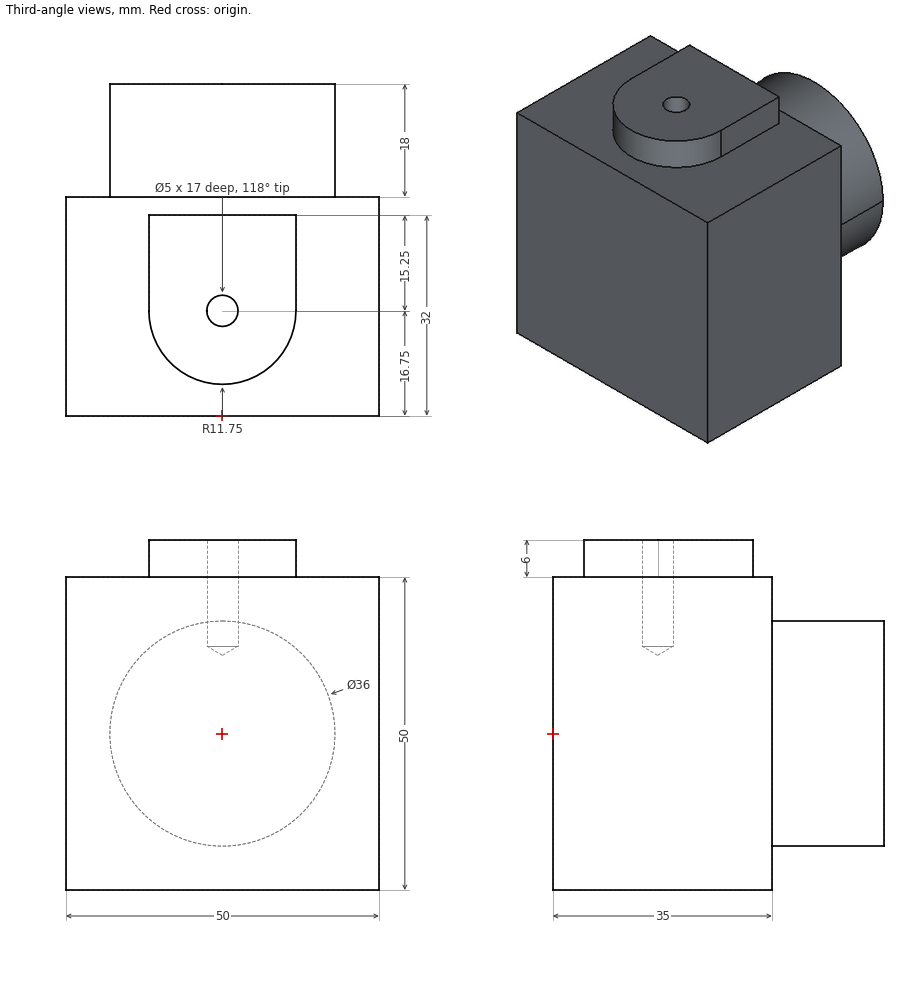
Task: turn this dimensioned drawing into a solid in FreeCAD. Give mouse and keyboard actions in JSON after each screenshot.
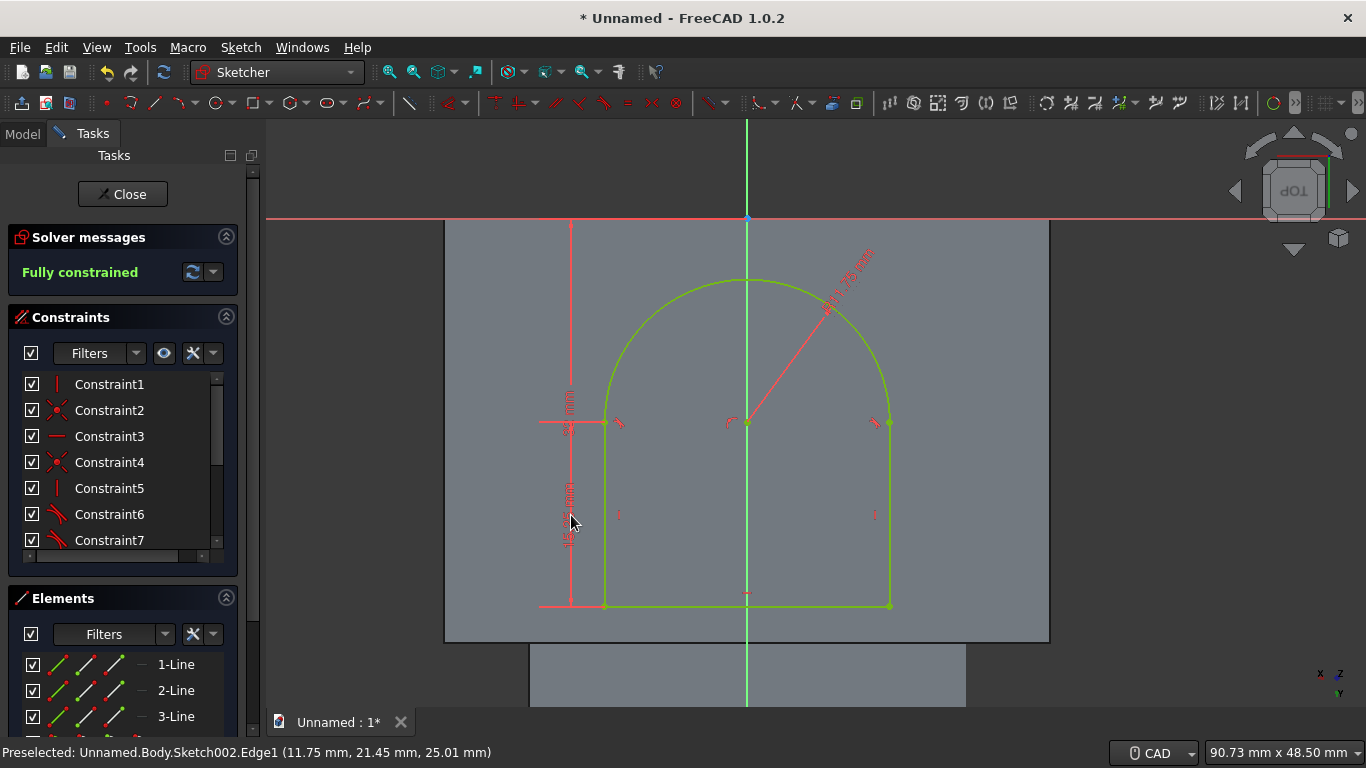
{"action": "left_click", "coordinate": [123, 194]}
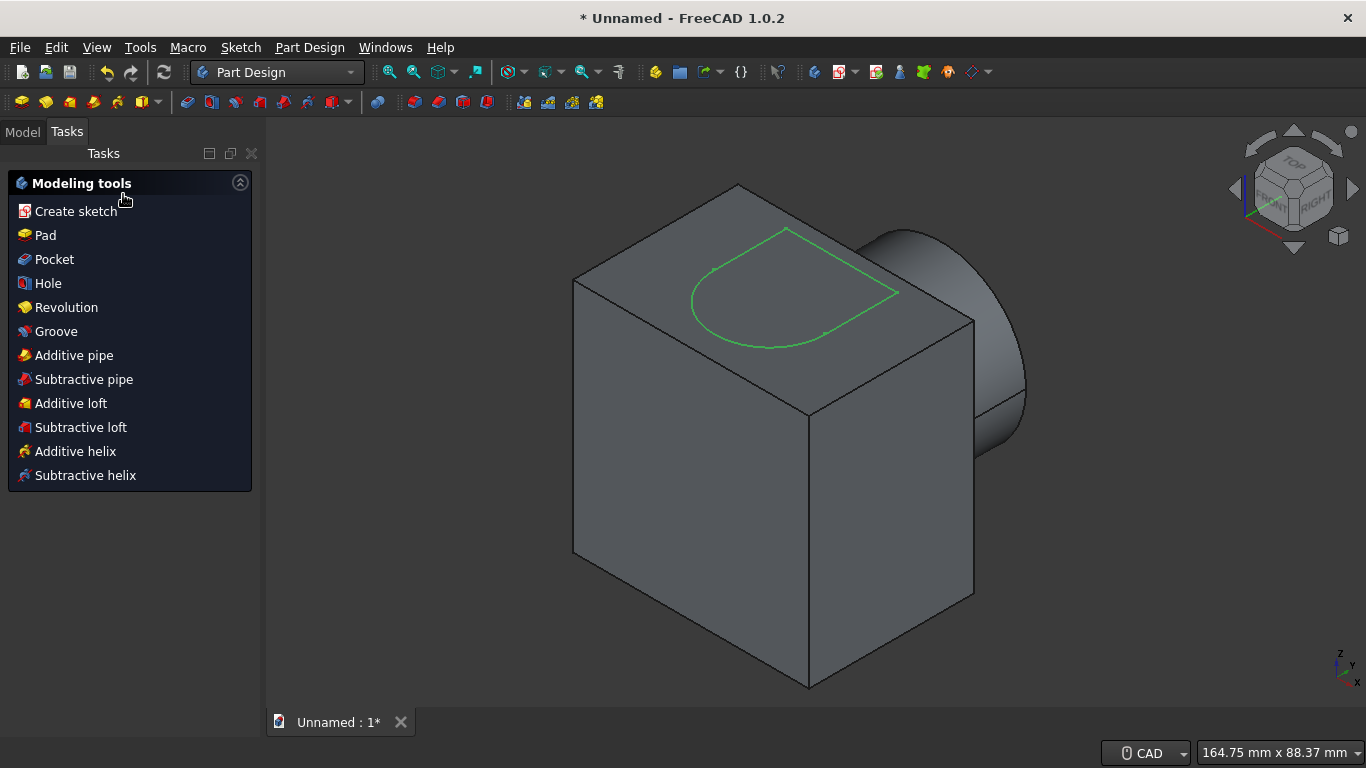
{"action": "left_click", "coordinate": [22, 102]}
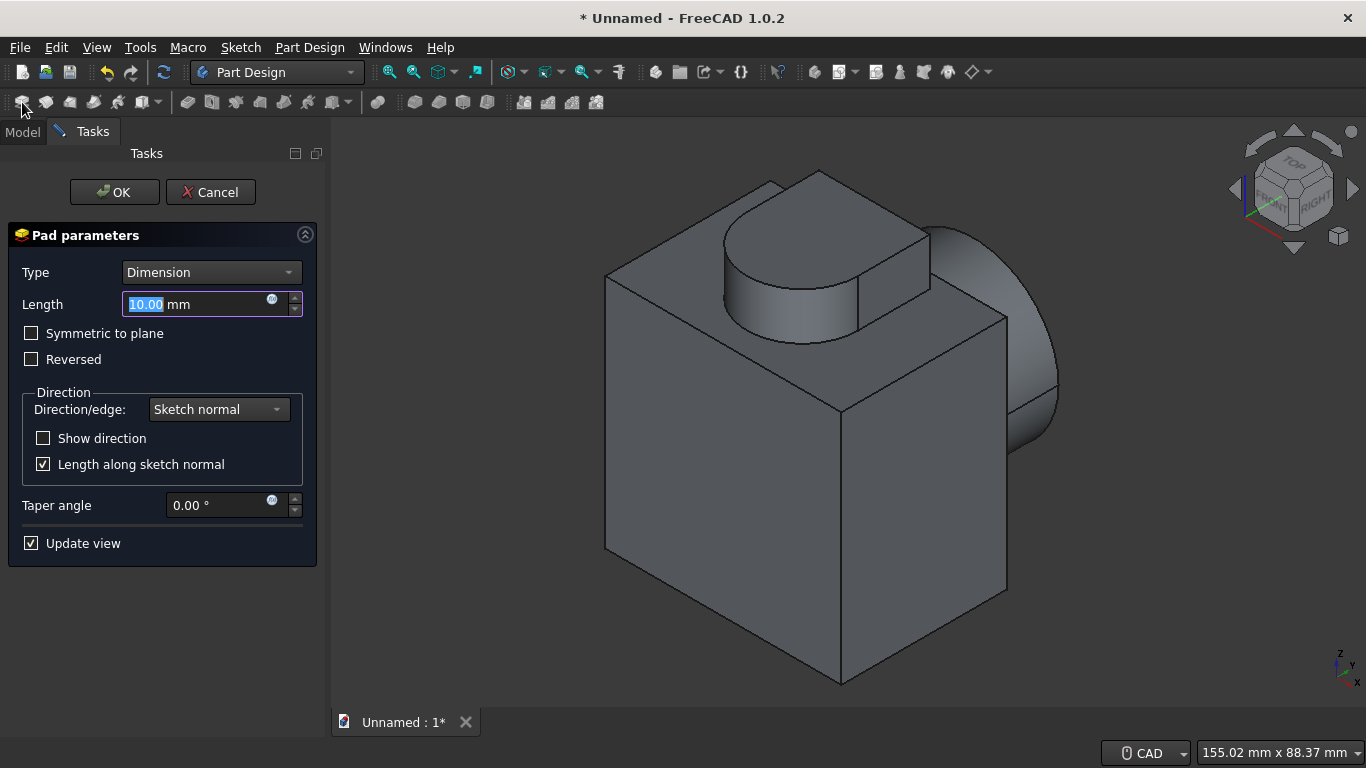
{"action": "type", "text": "6"}
{"action": "key", "text": "Tab"}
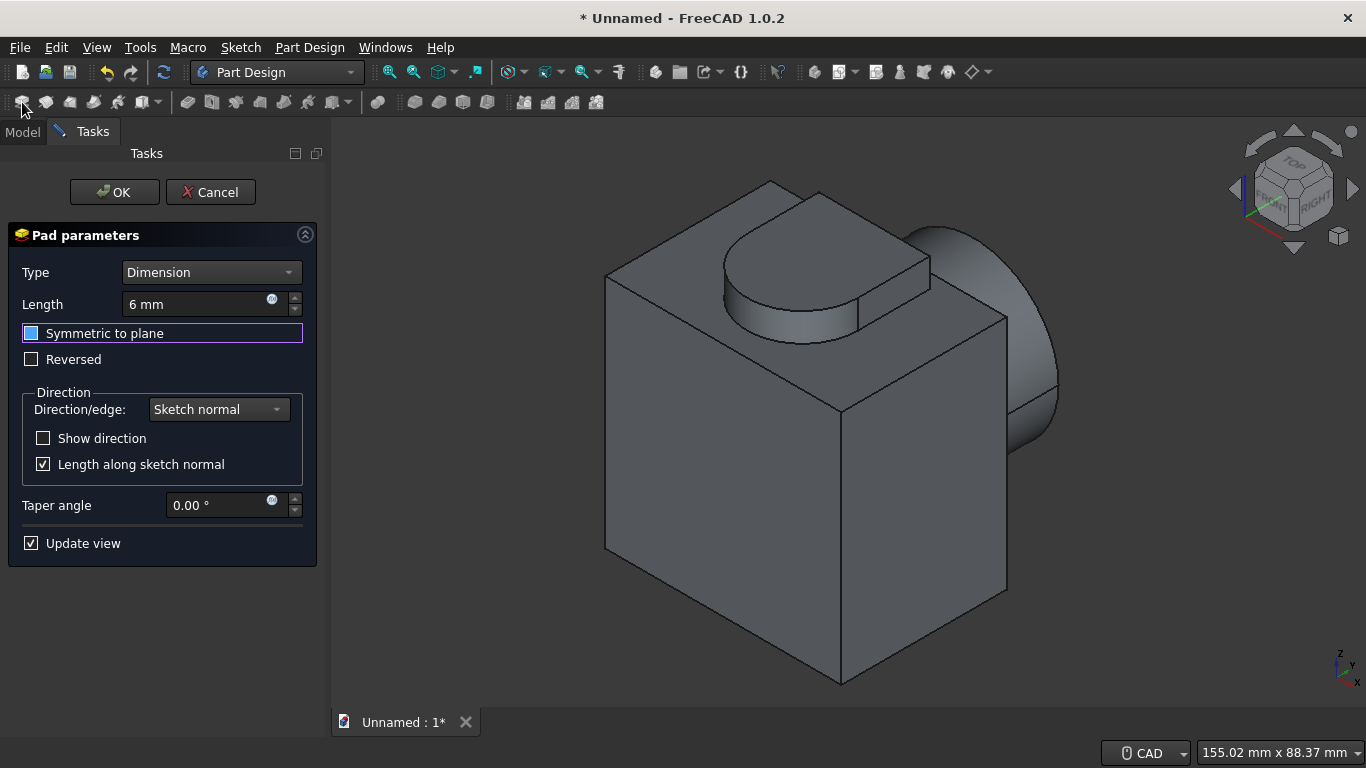
{"action": "left_click", "coordinate": [115, 192]}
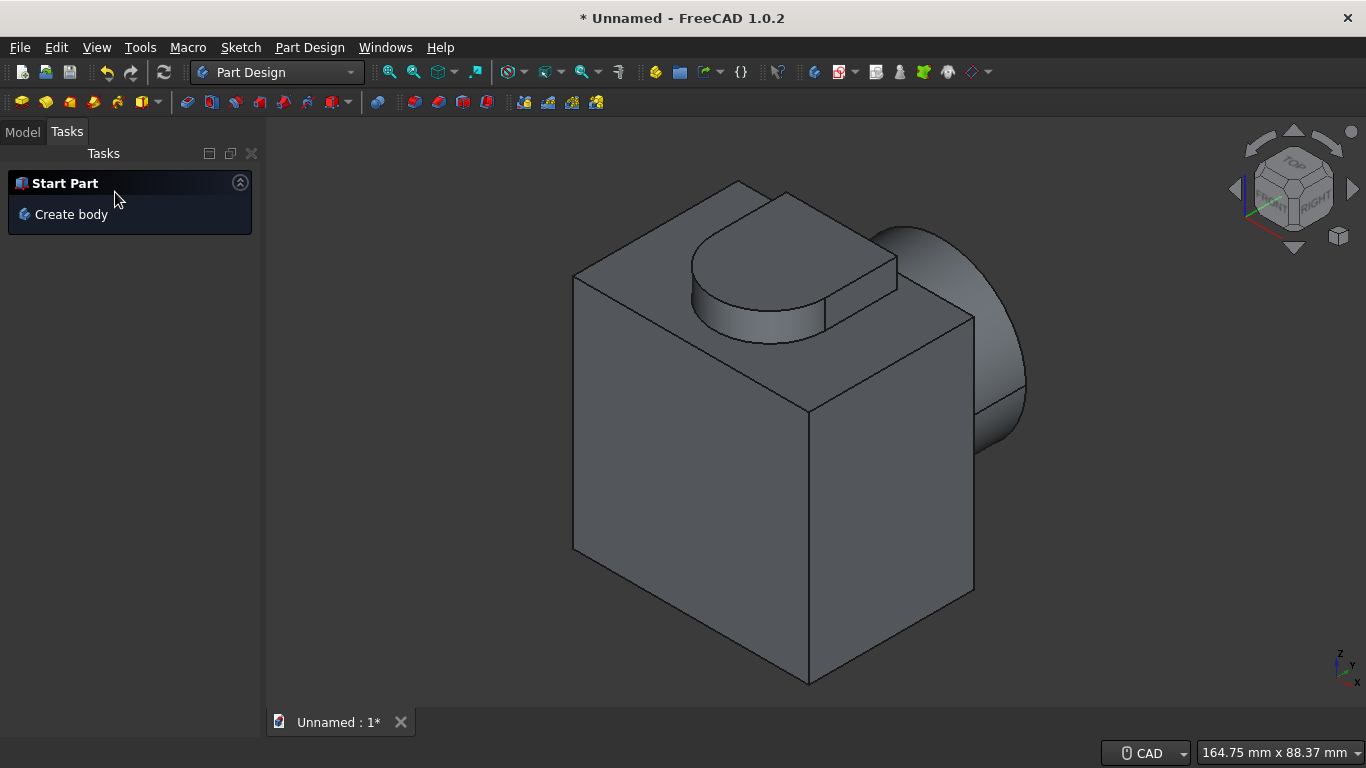
{"action": "left_click", "coordinate": [390, 72]}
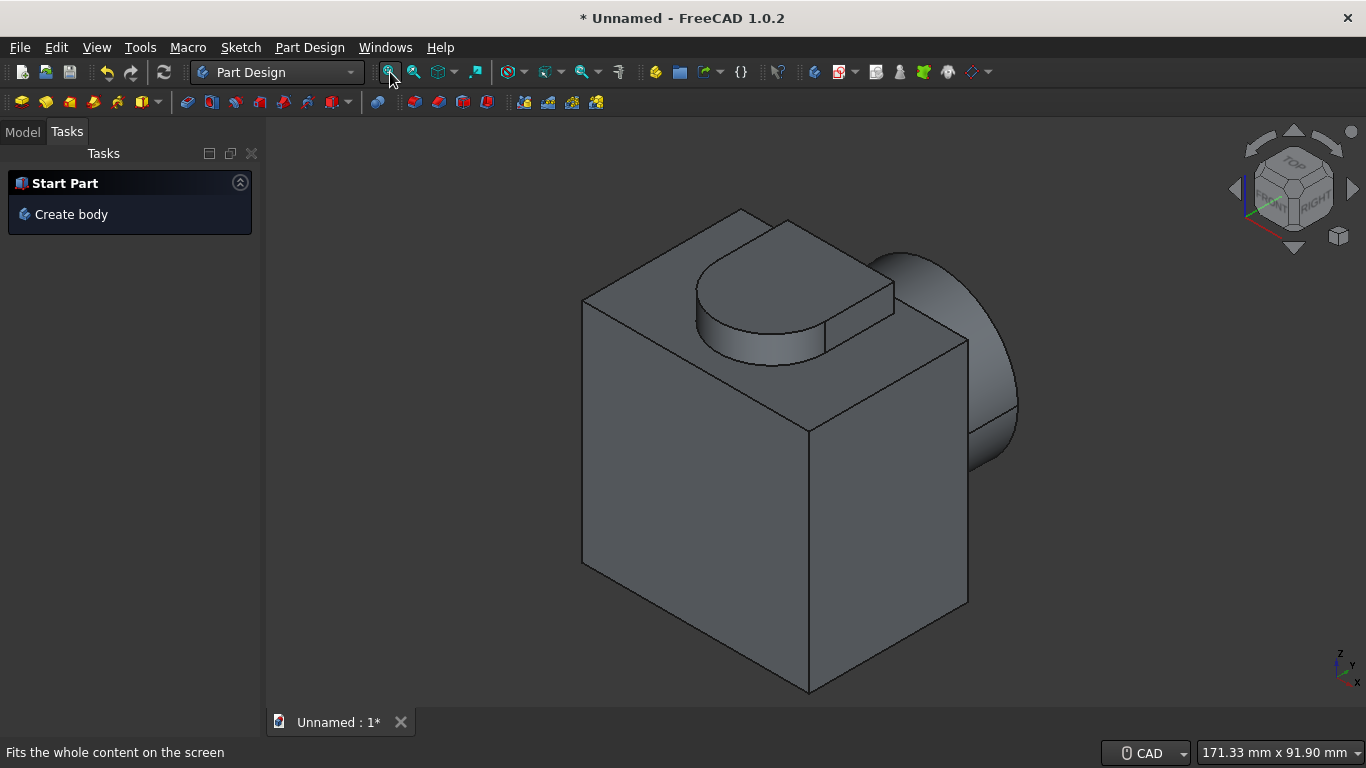
{"action": "left_click", "coordinate": [780, 285]}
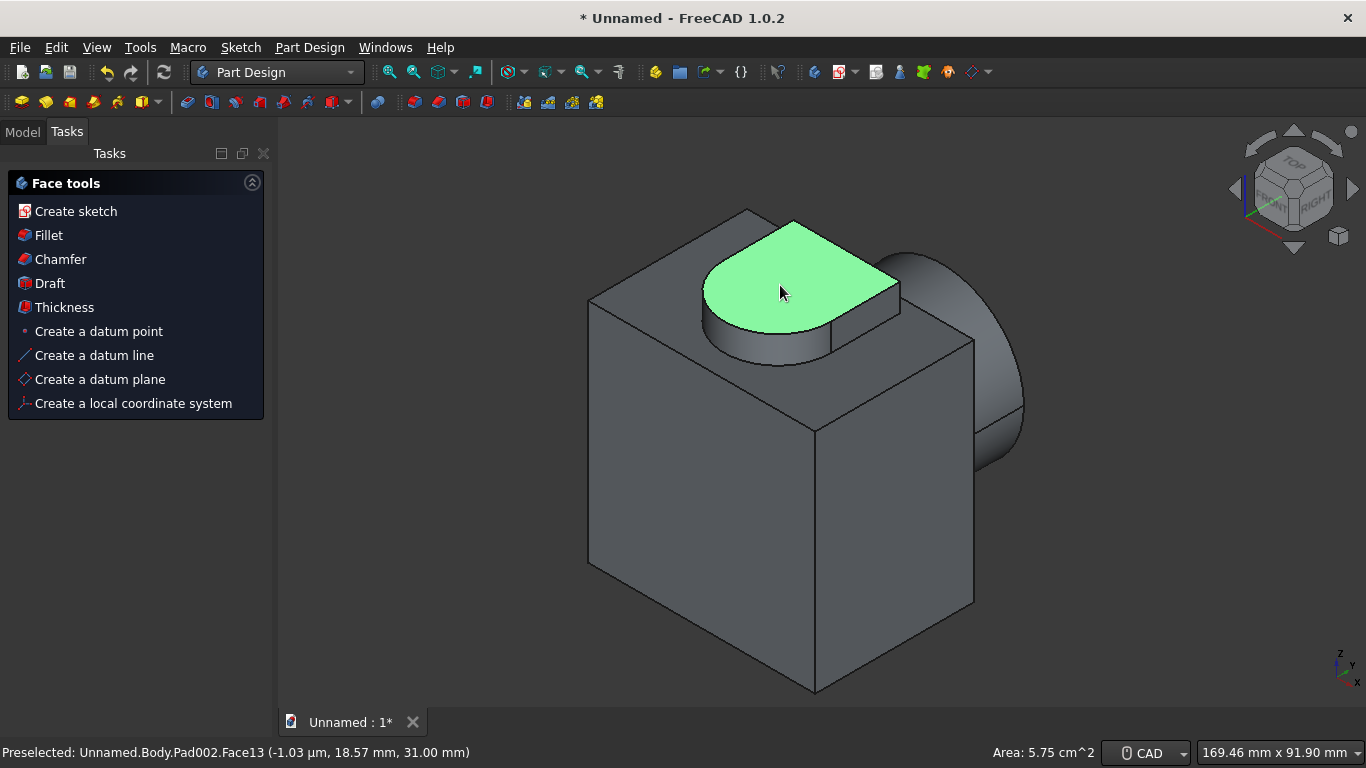
{"action": "left_click", "coordinate": [840, 72]}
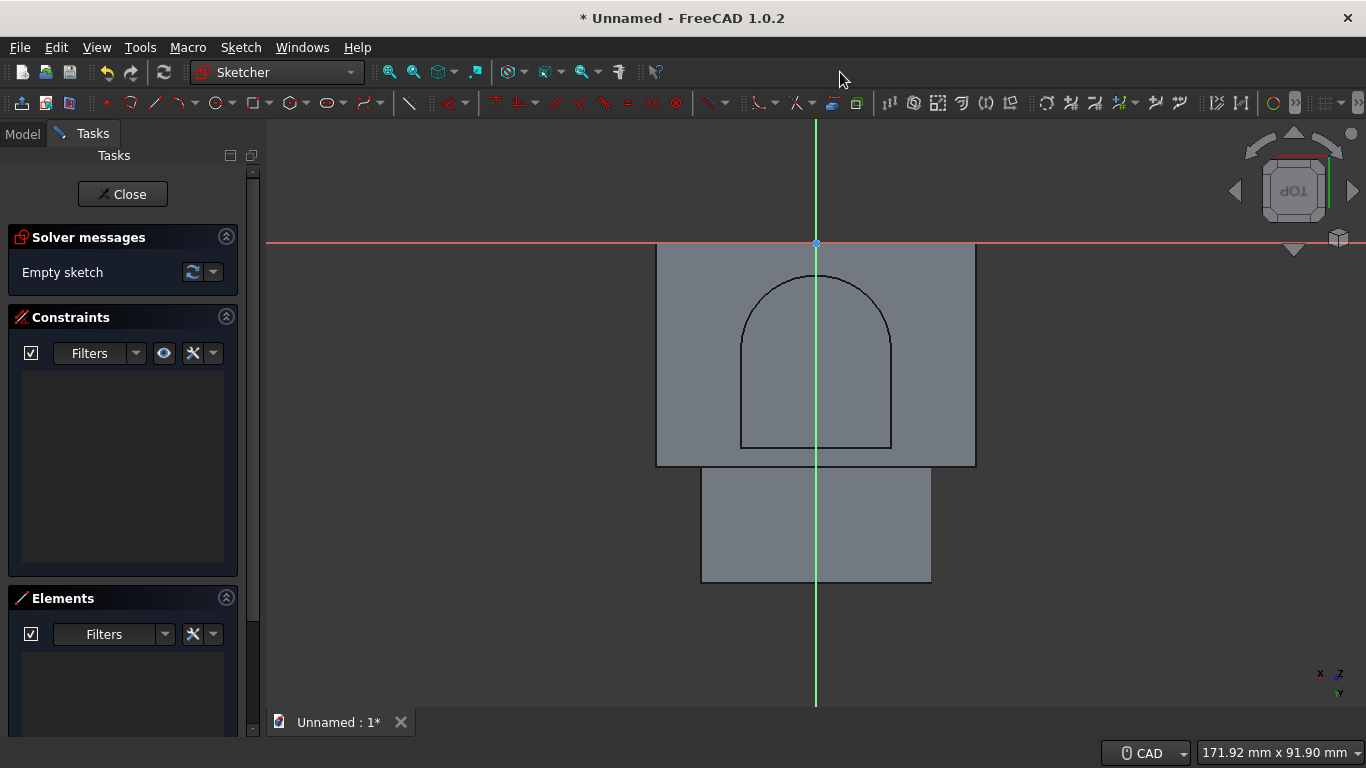
{"action": "scroll", "coordinate": [823, 344], "scroll_direction": "up", "scroll_amount": 12}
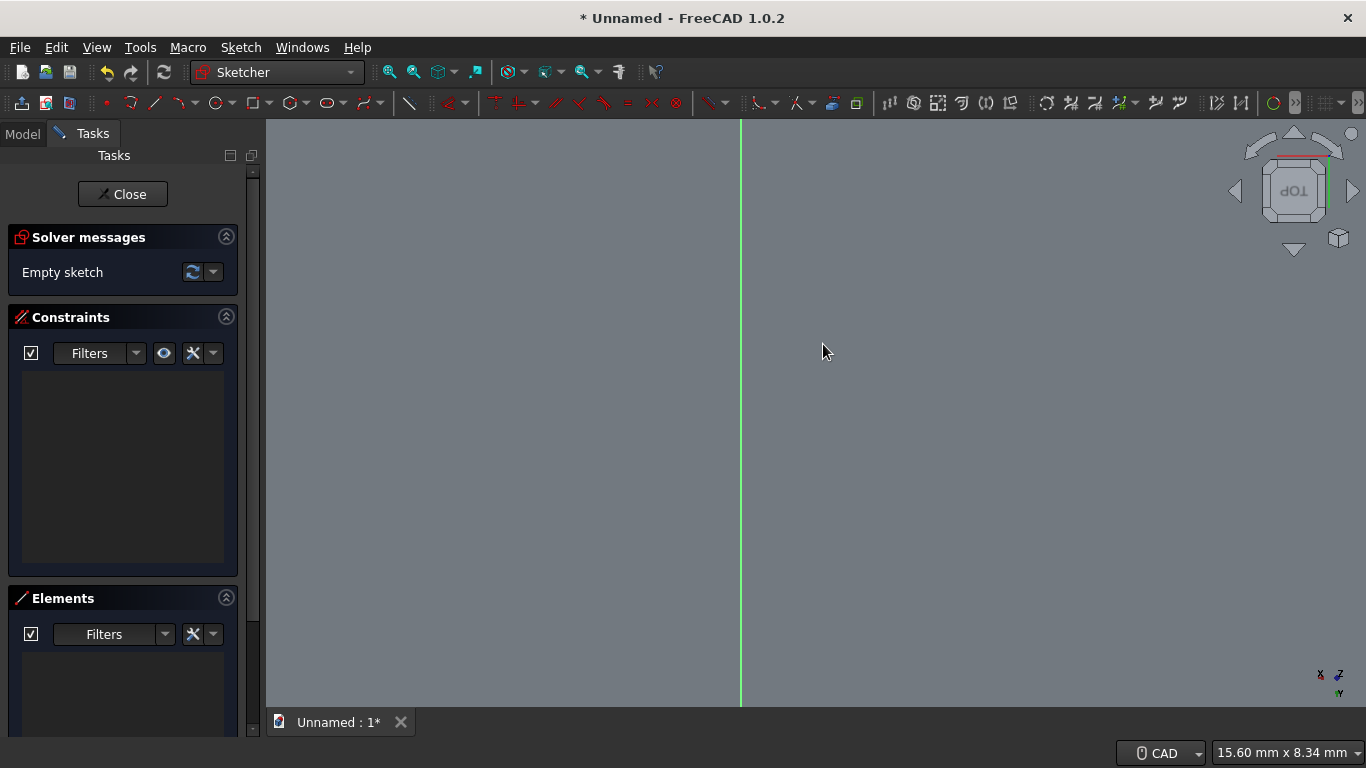
{"action": "key", "text": "g c"}